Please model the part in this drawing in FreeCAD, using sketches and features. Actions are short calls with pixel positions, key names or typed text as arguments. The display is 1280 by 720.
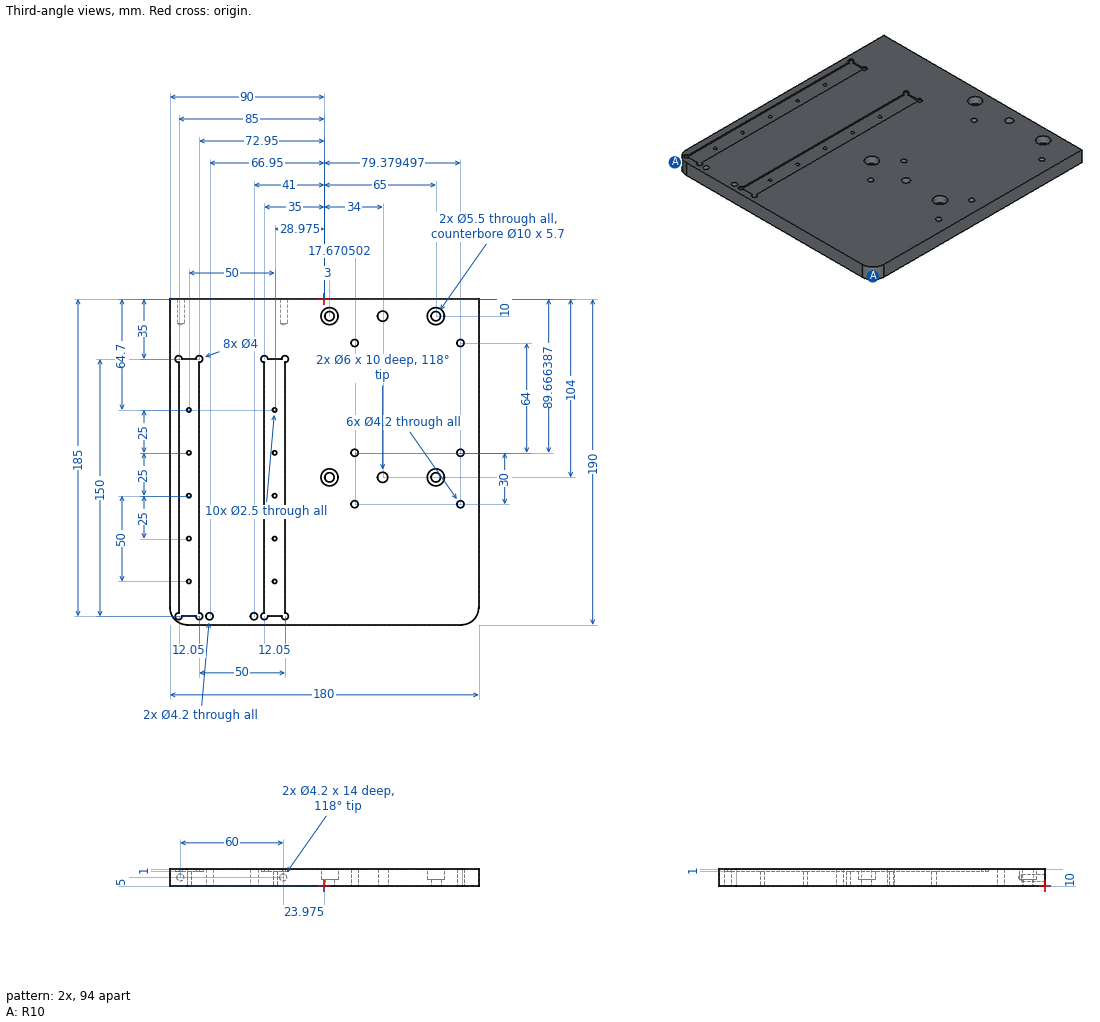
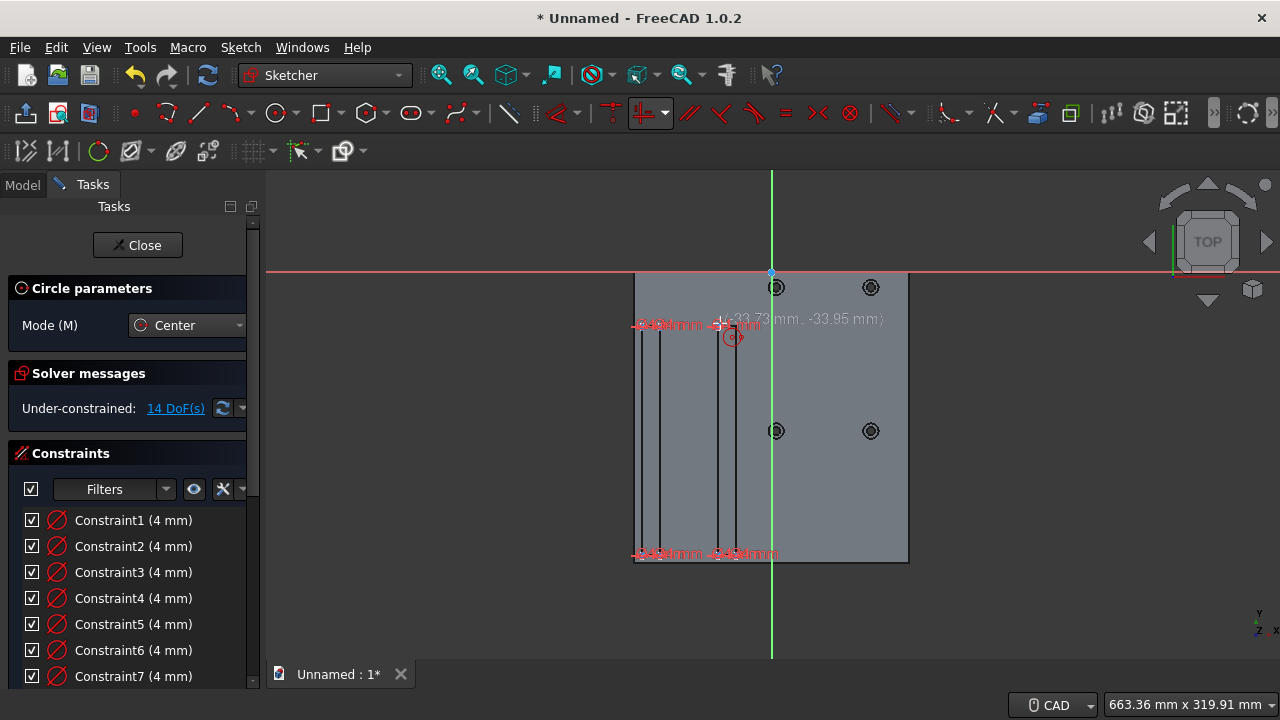
scroll(736, 326, up, 11)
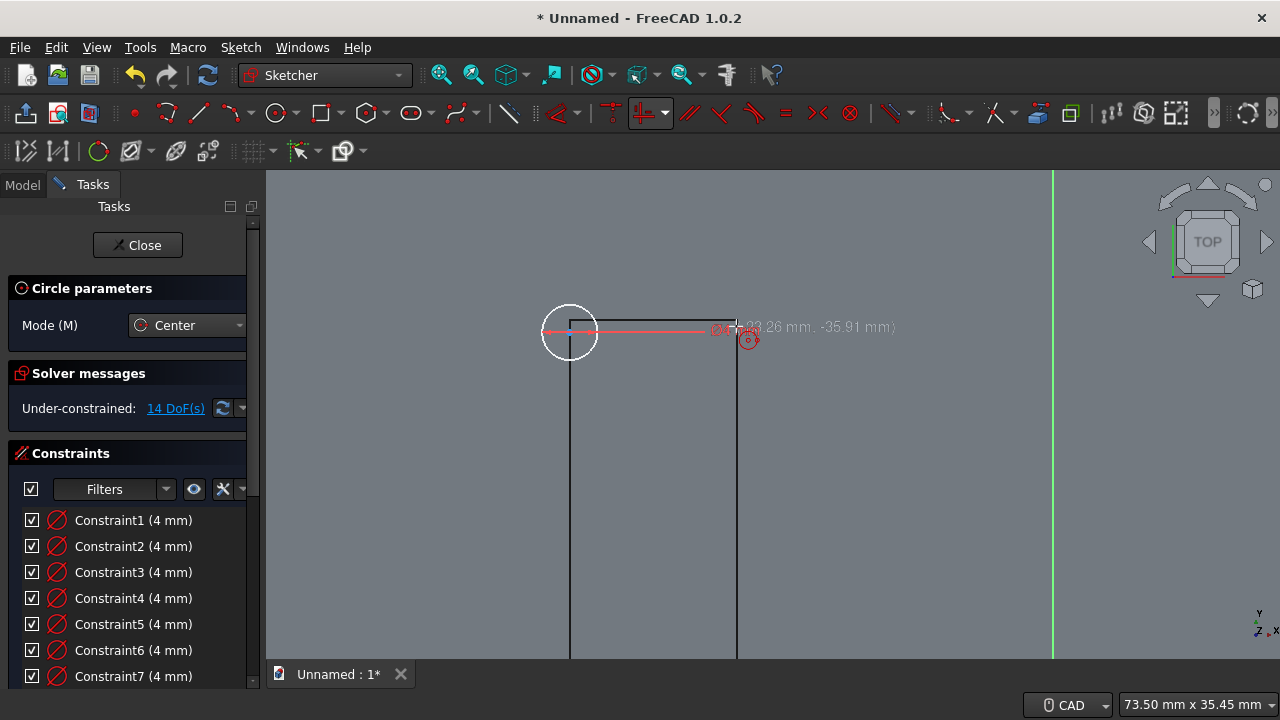
scroll(736, 326, down, 11)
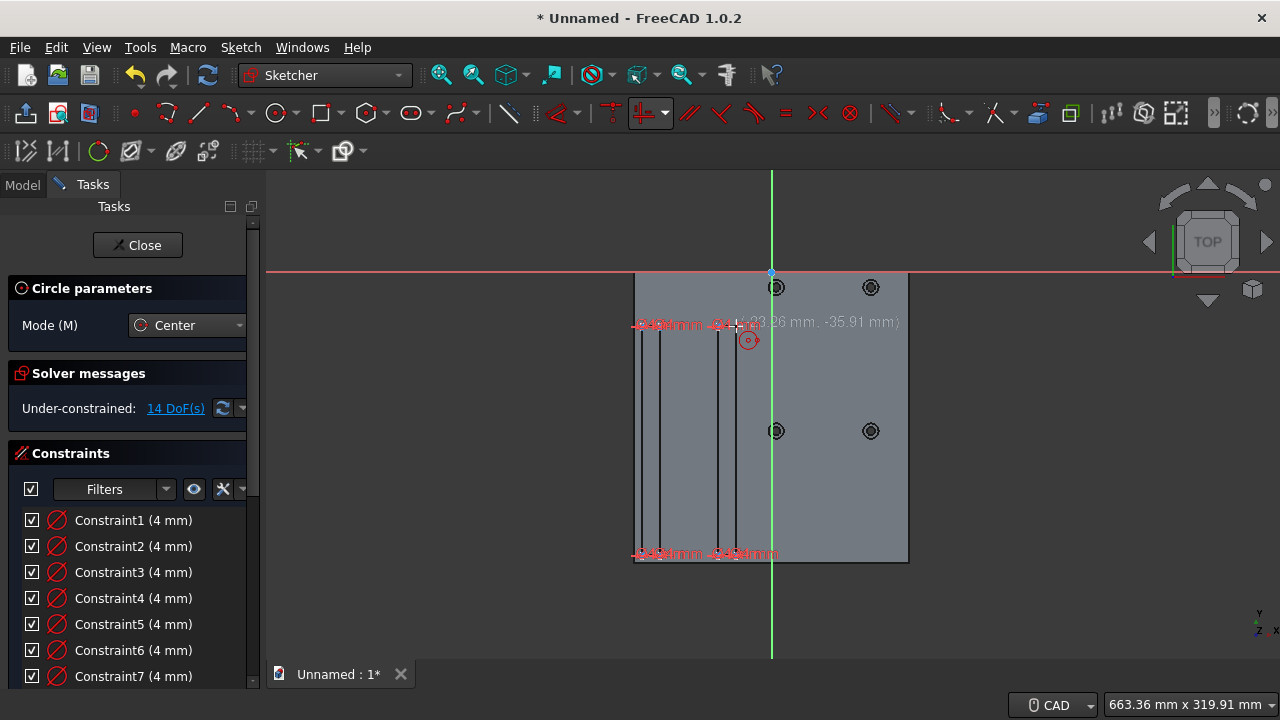
click(736, 326)
move(739, 323)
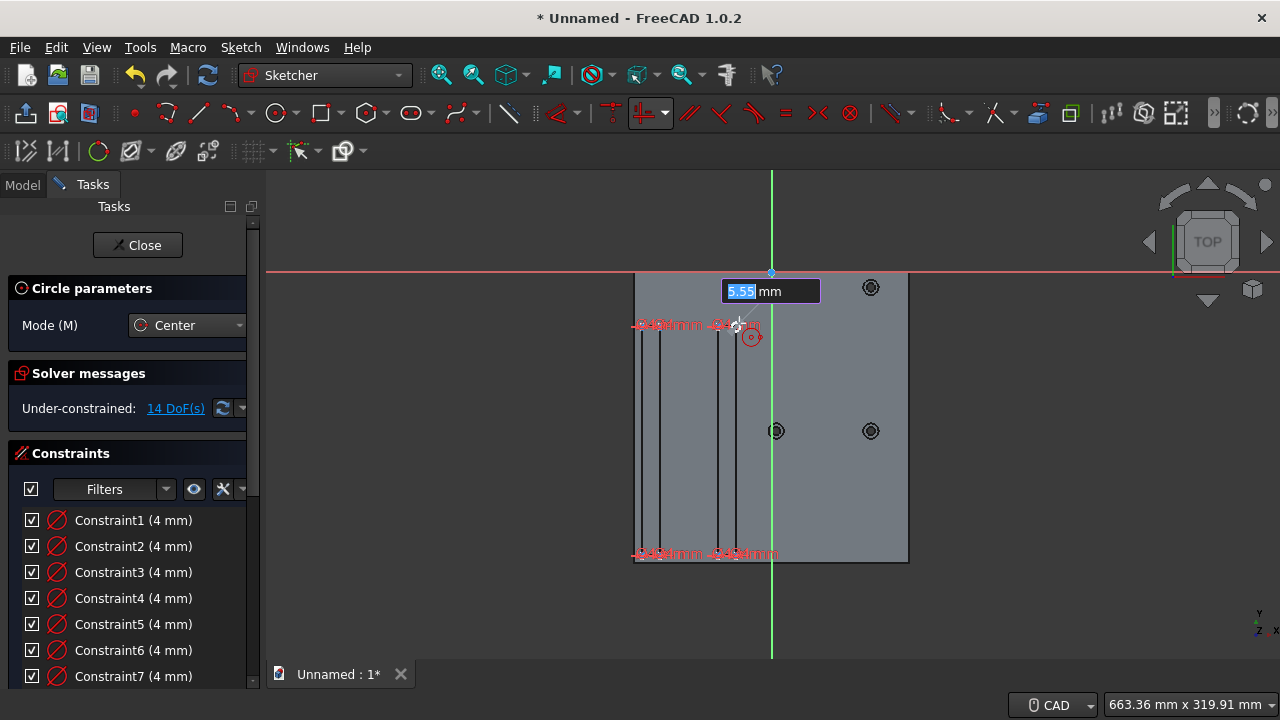
text(4)
key(Return)
key(Escape)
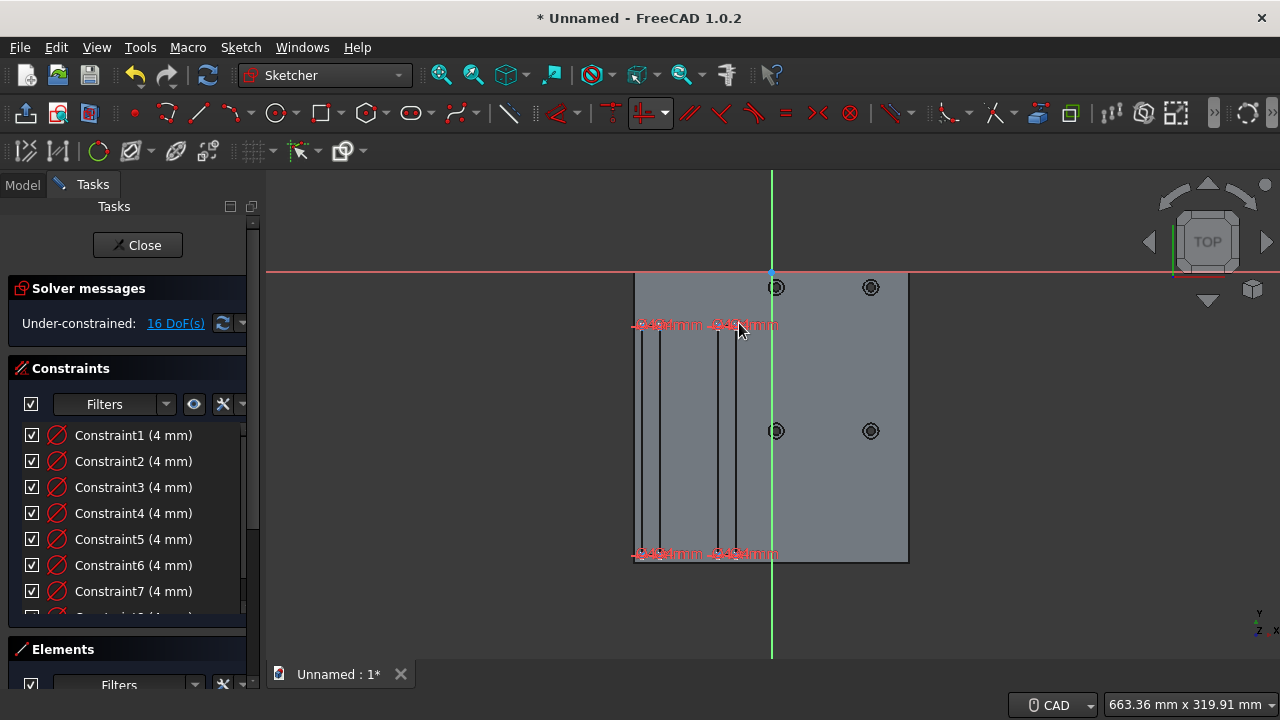
click(660, 327)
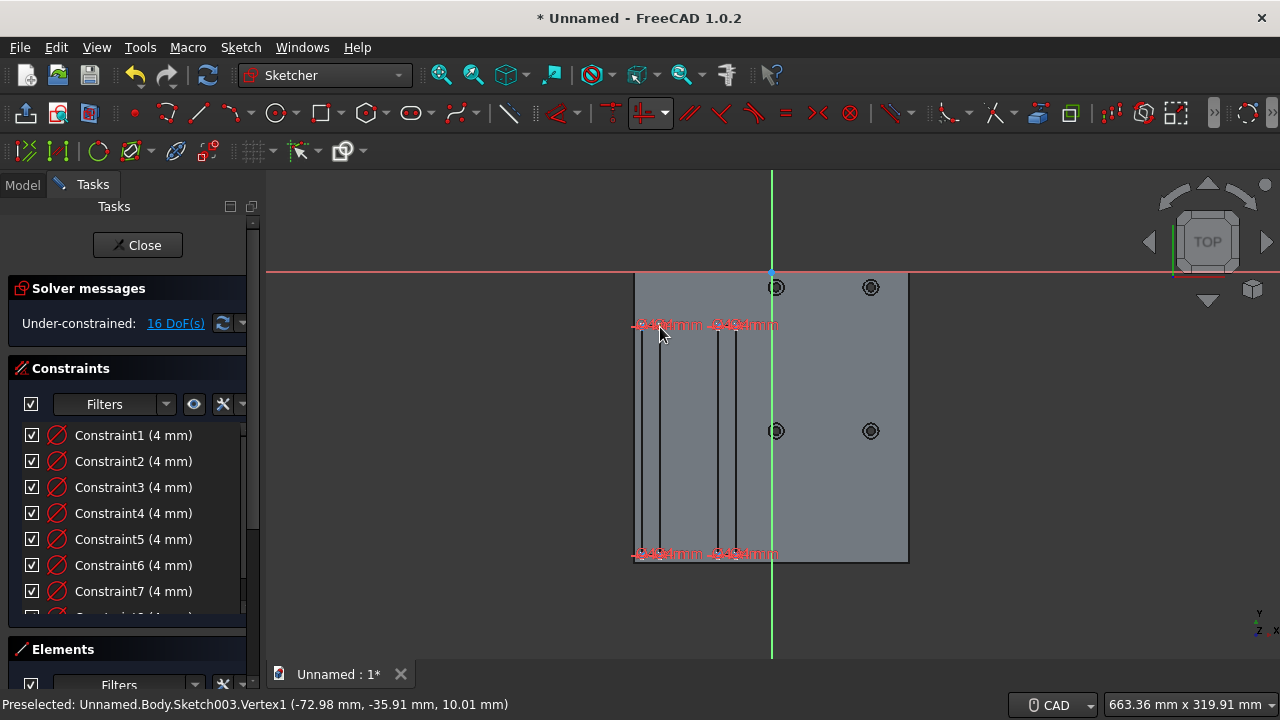
click(642, 327)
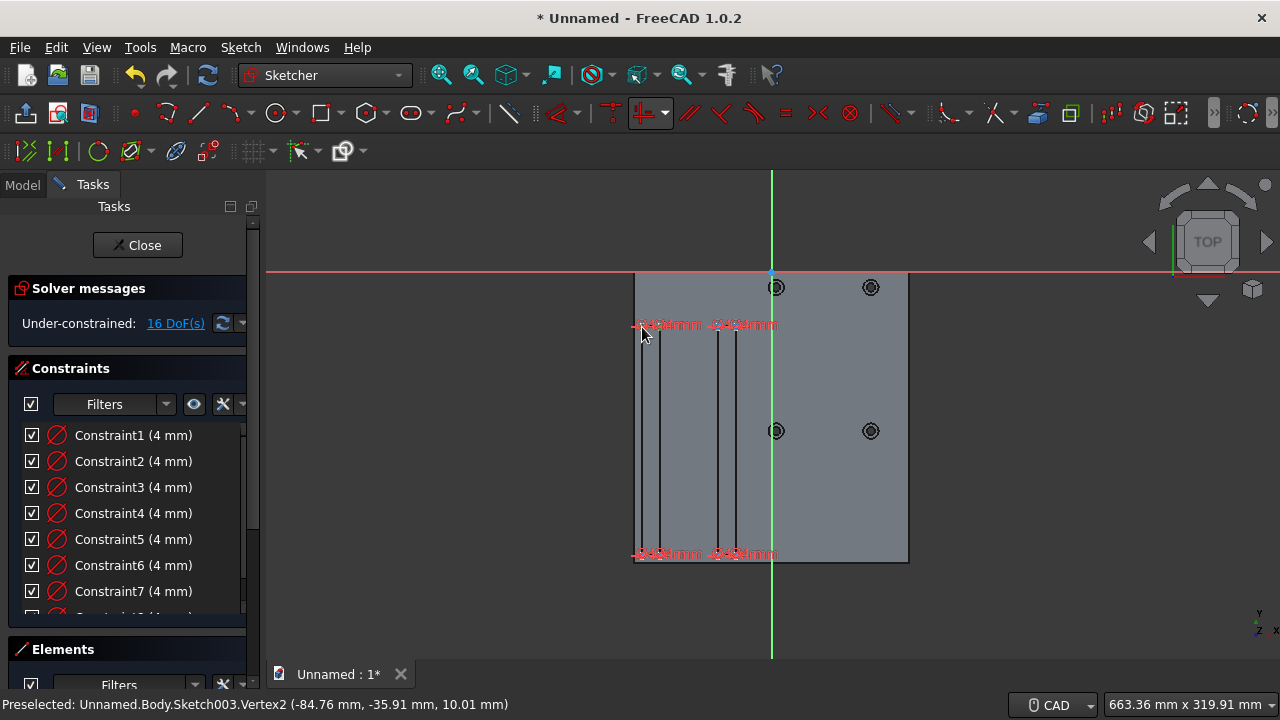
key(h)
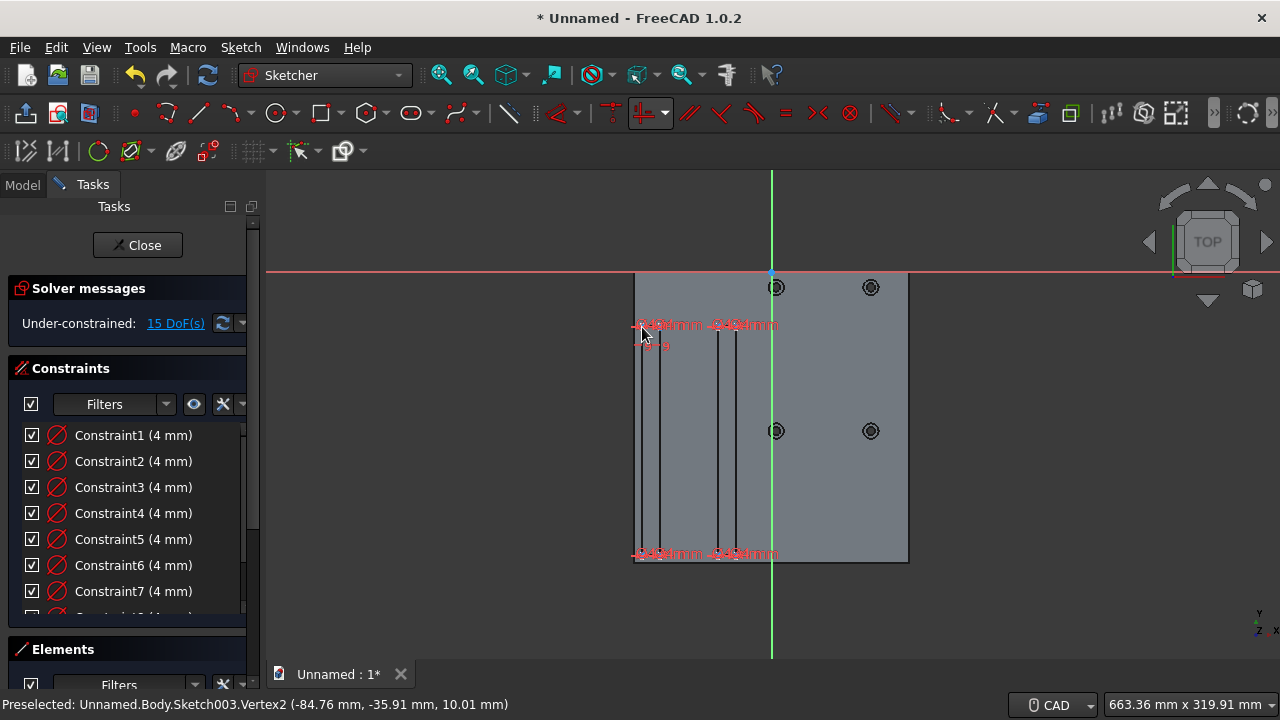
click(642, 327)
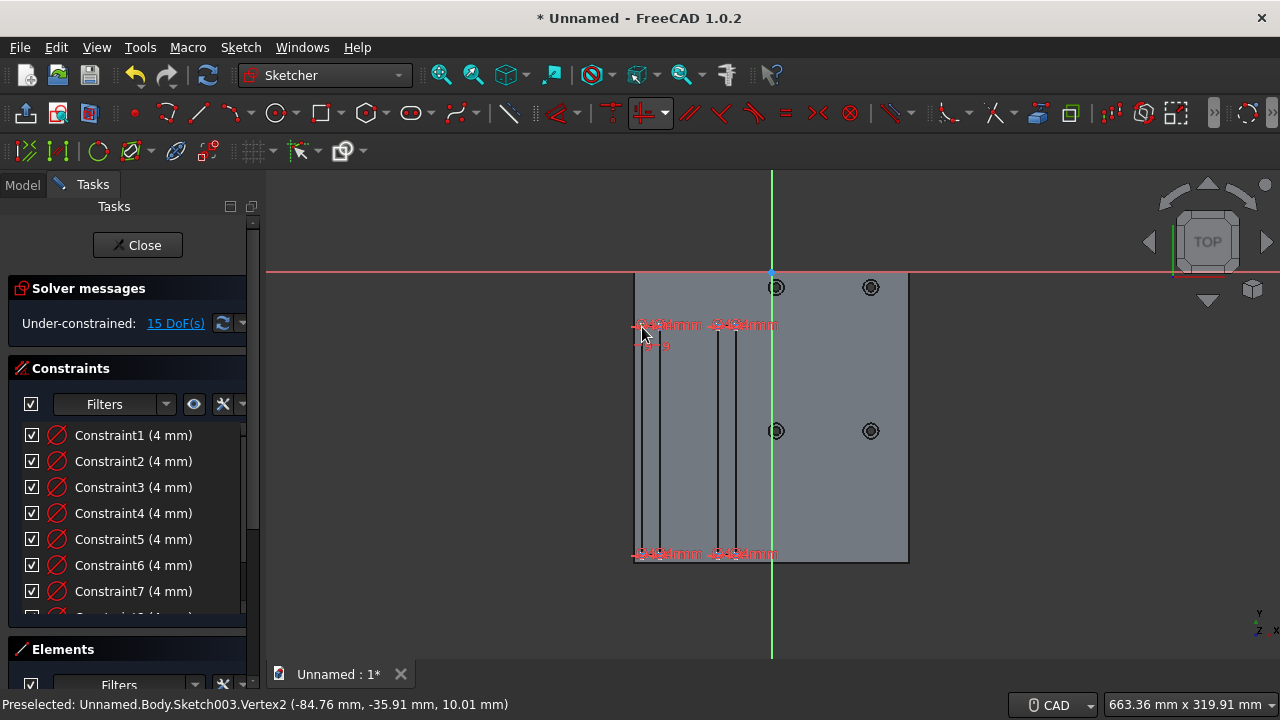
click(642, 556)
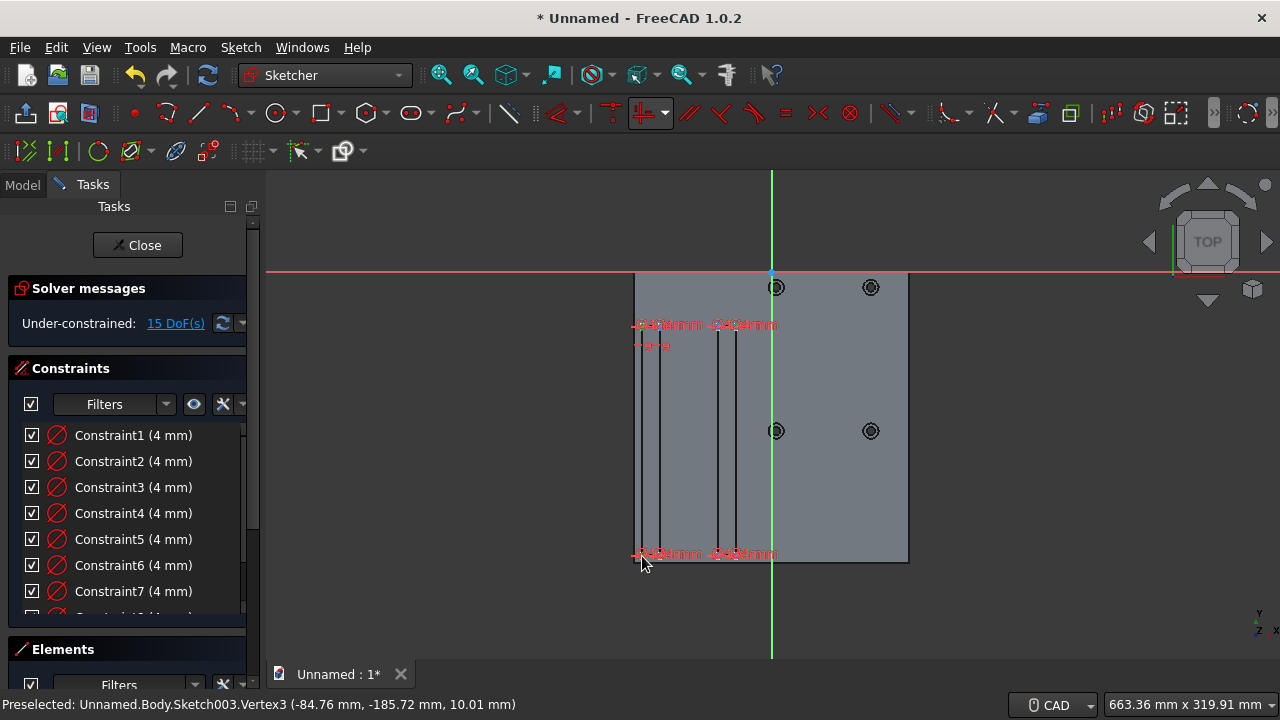
key(v)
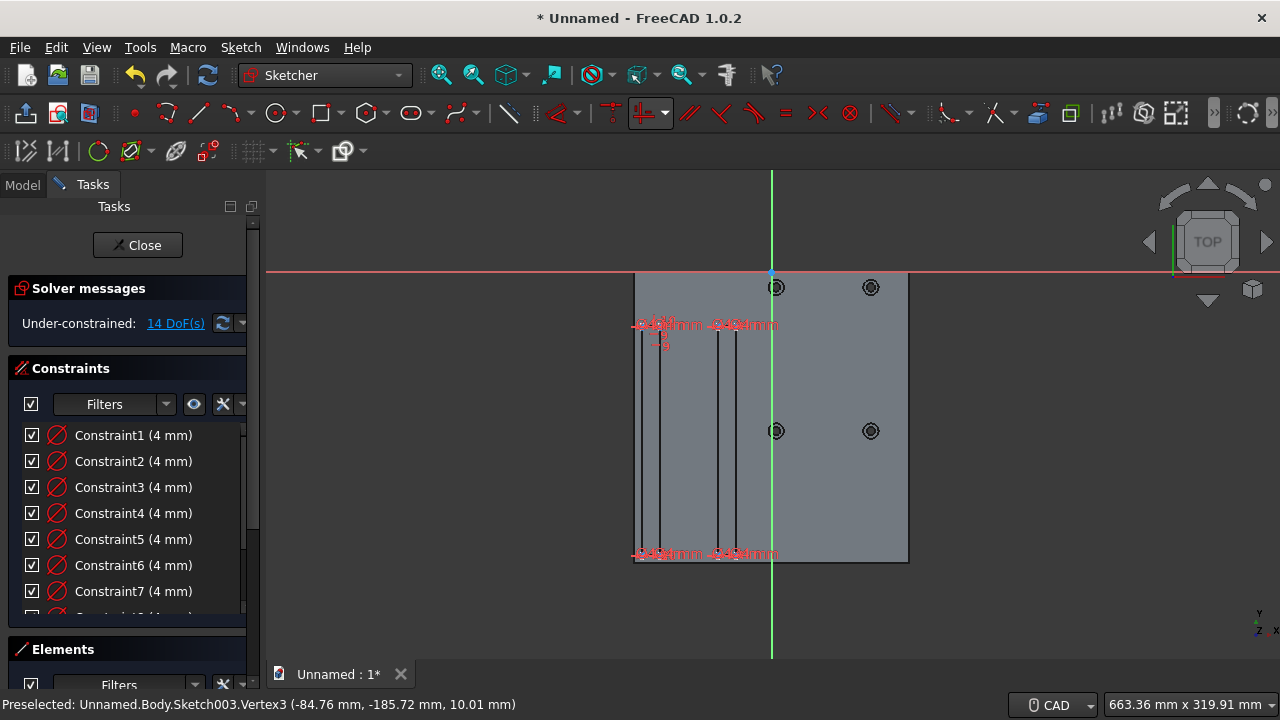
click(660, 327)